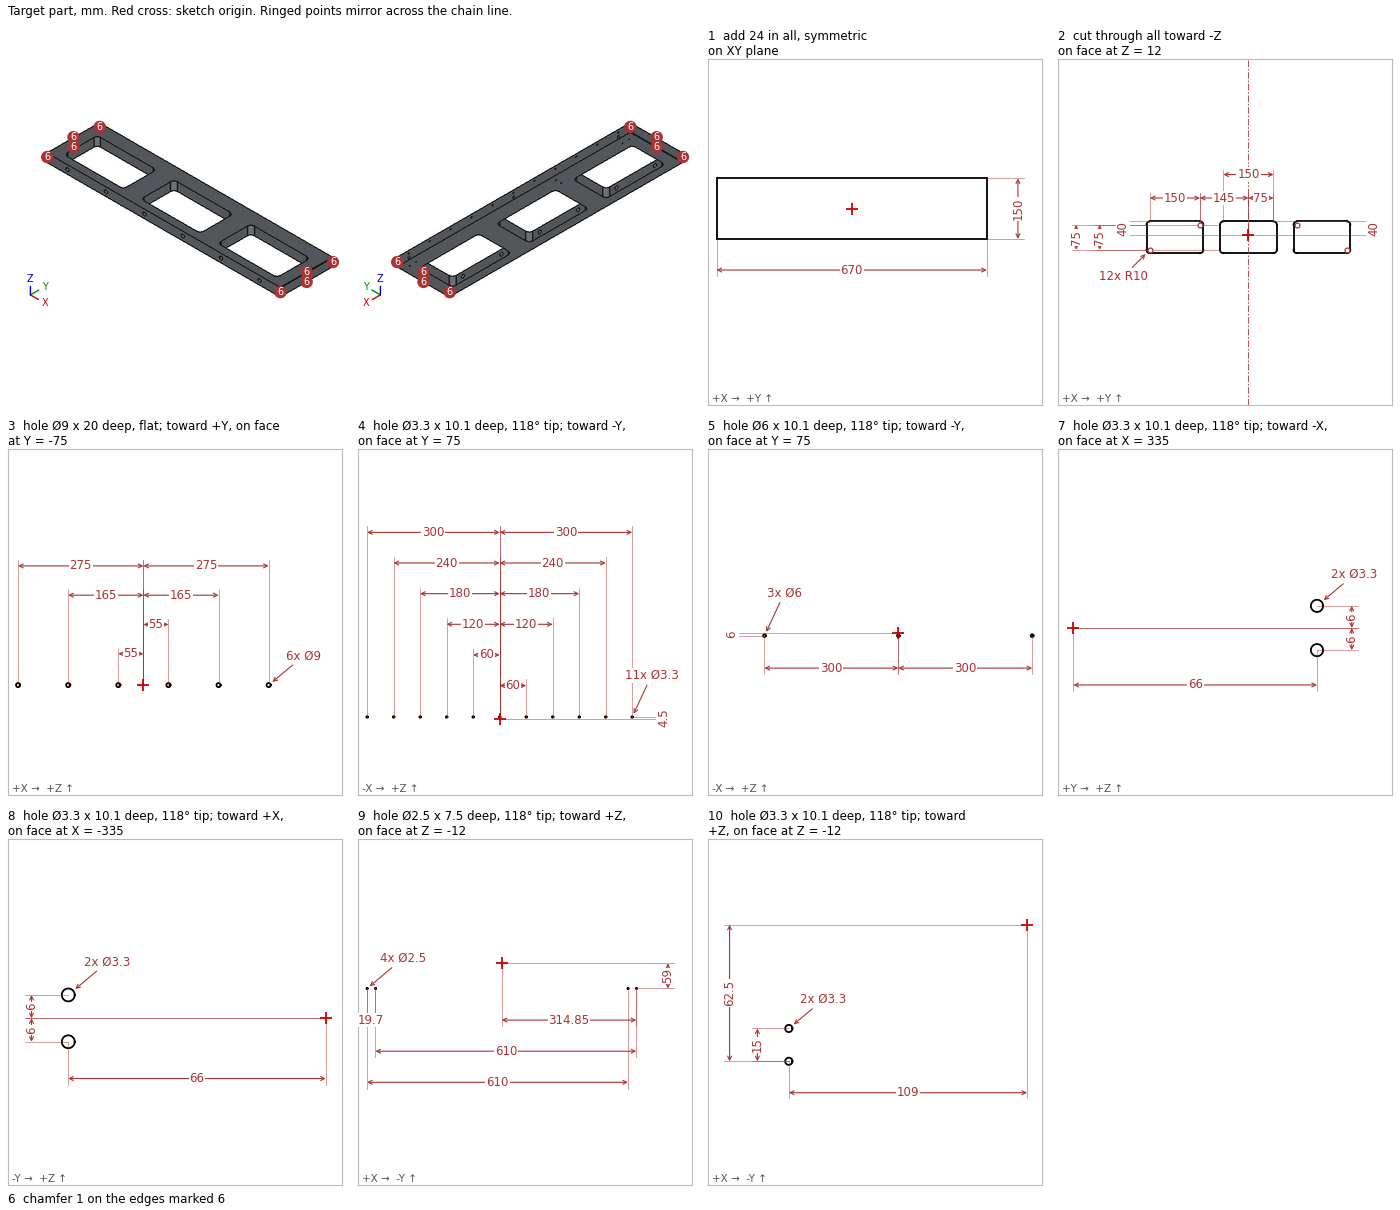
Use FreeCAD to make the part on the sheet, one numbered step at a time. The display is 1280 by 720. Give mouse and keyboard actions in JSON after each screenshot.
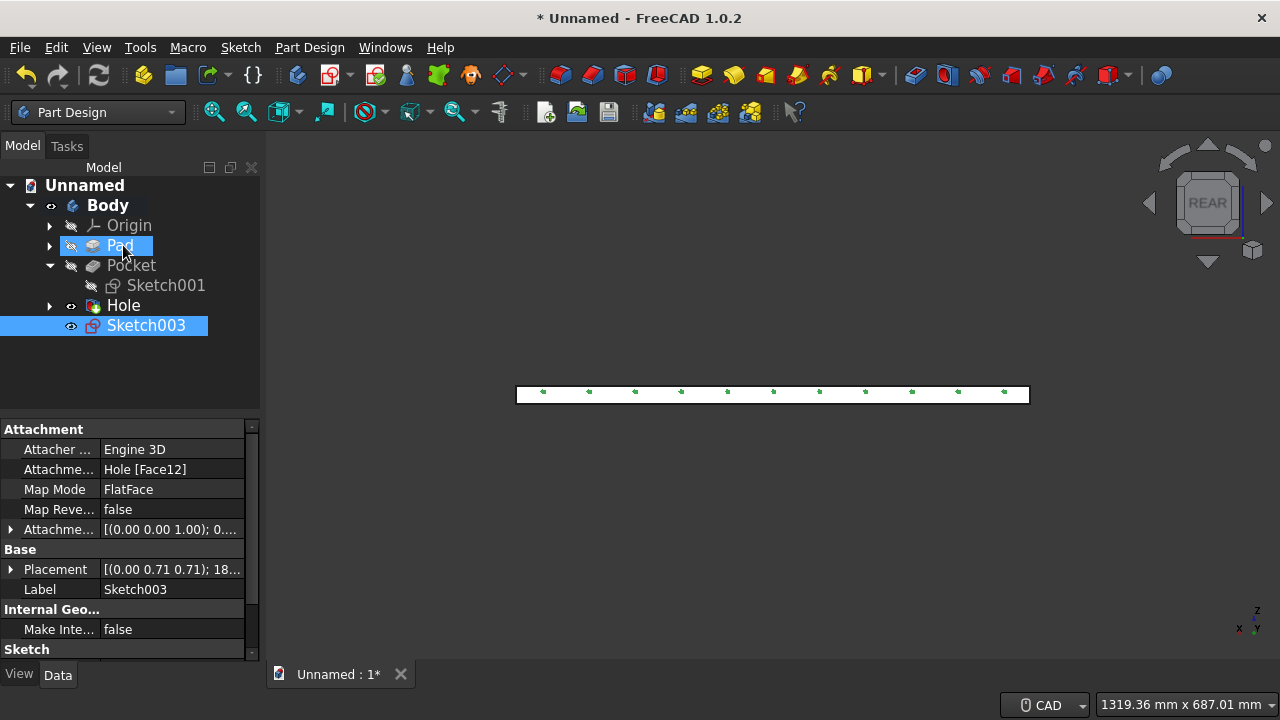
{"action": "left_click", "coordinate": [948, 76]}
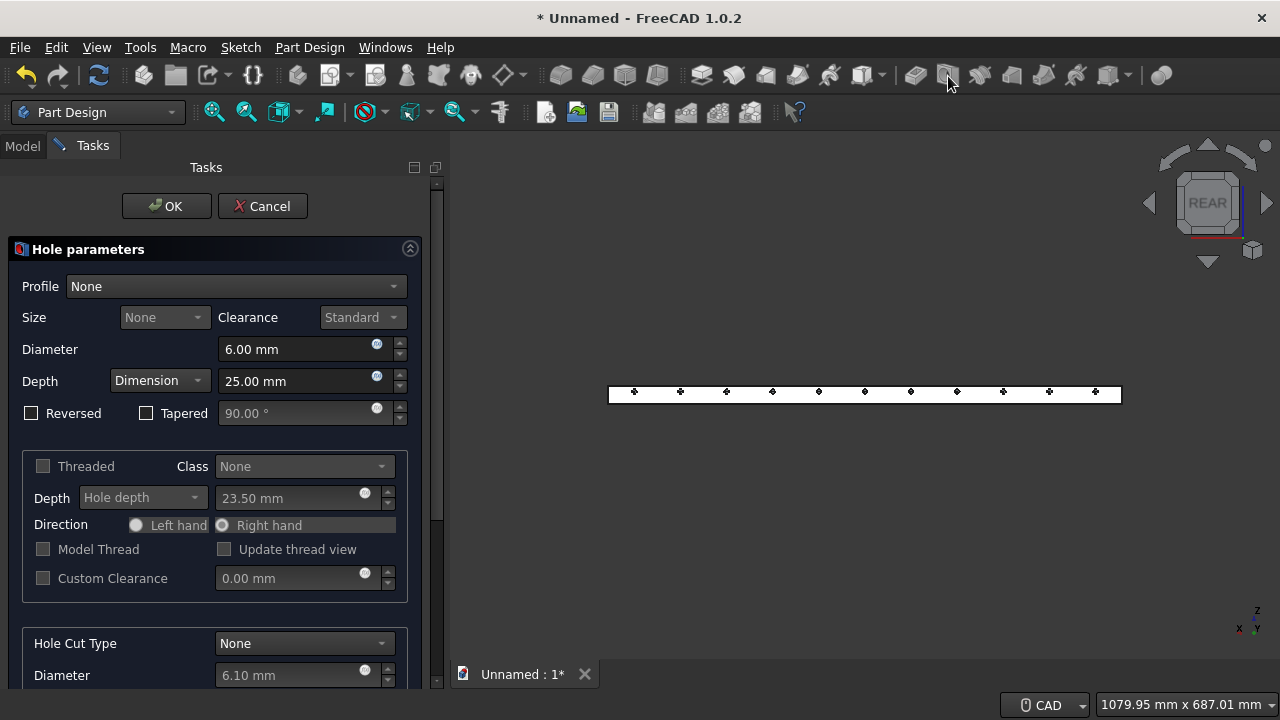
{"action": "triple_click", "coordinate": [305, 349]}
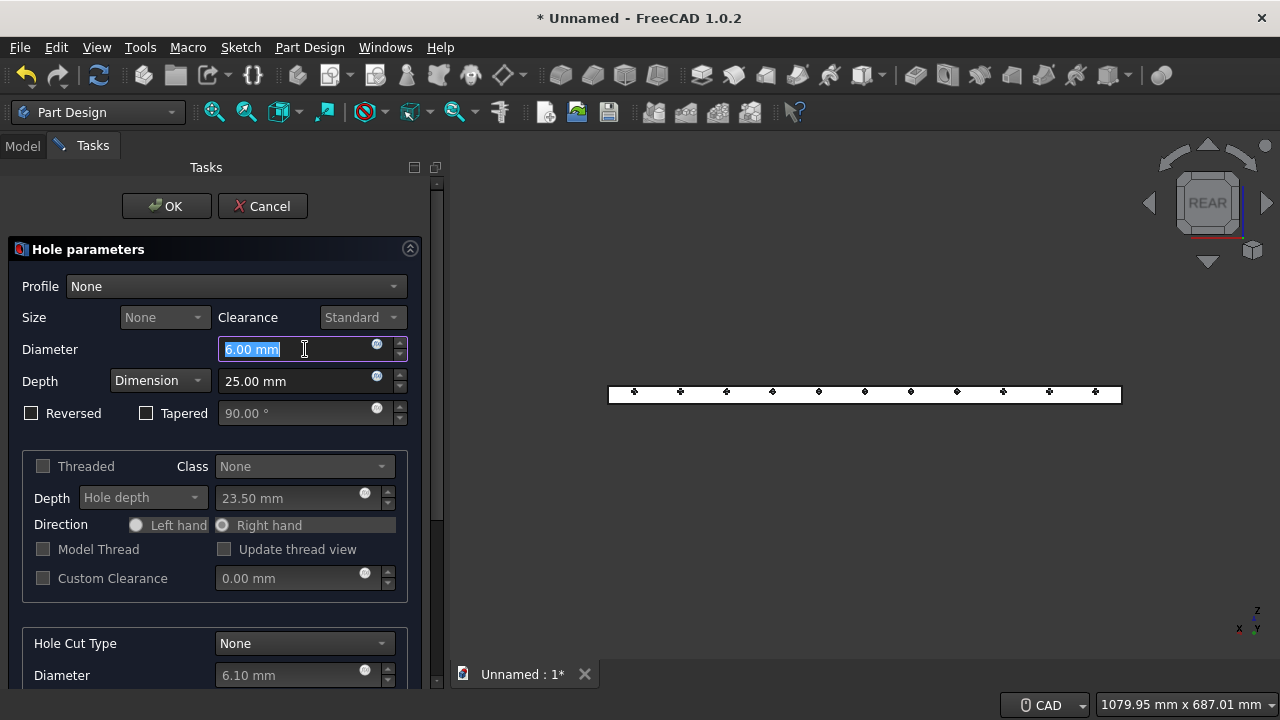
{"action": "type", "text": "3.3"}
{"action": "key", "text": "Tab"}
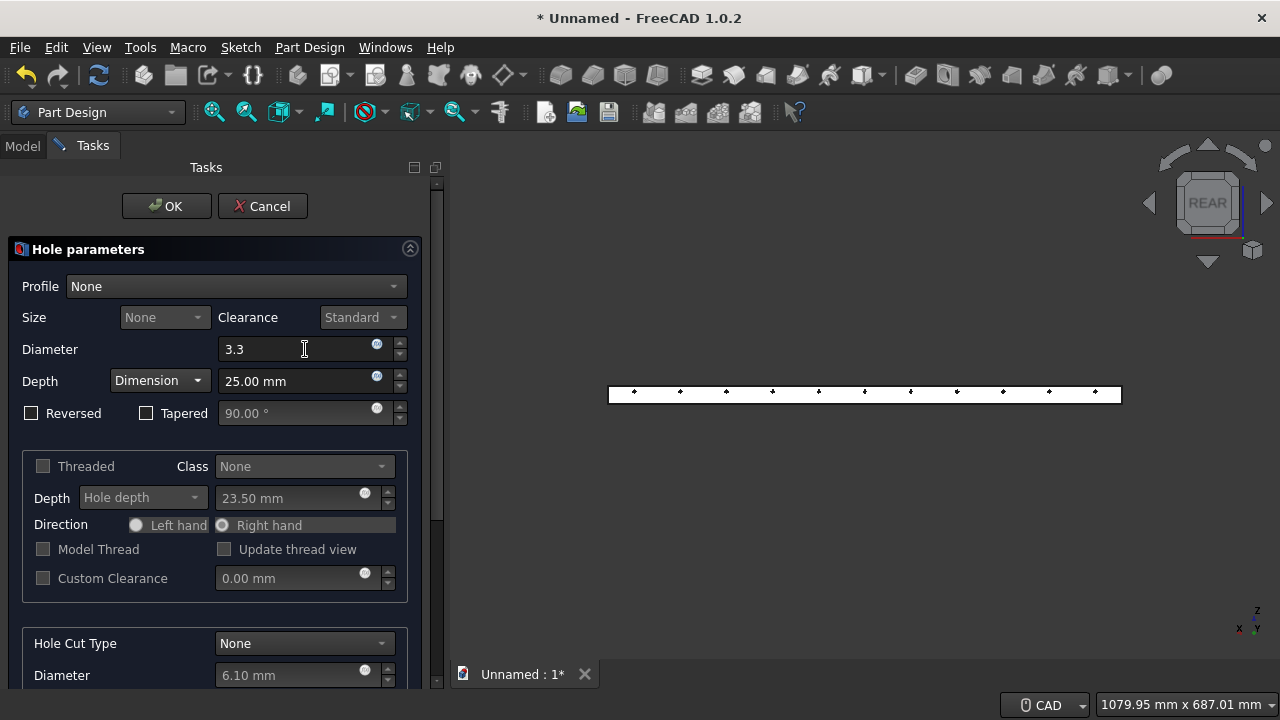
{"action": "triple_click", "coordinate": [305, 381]}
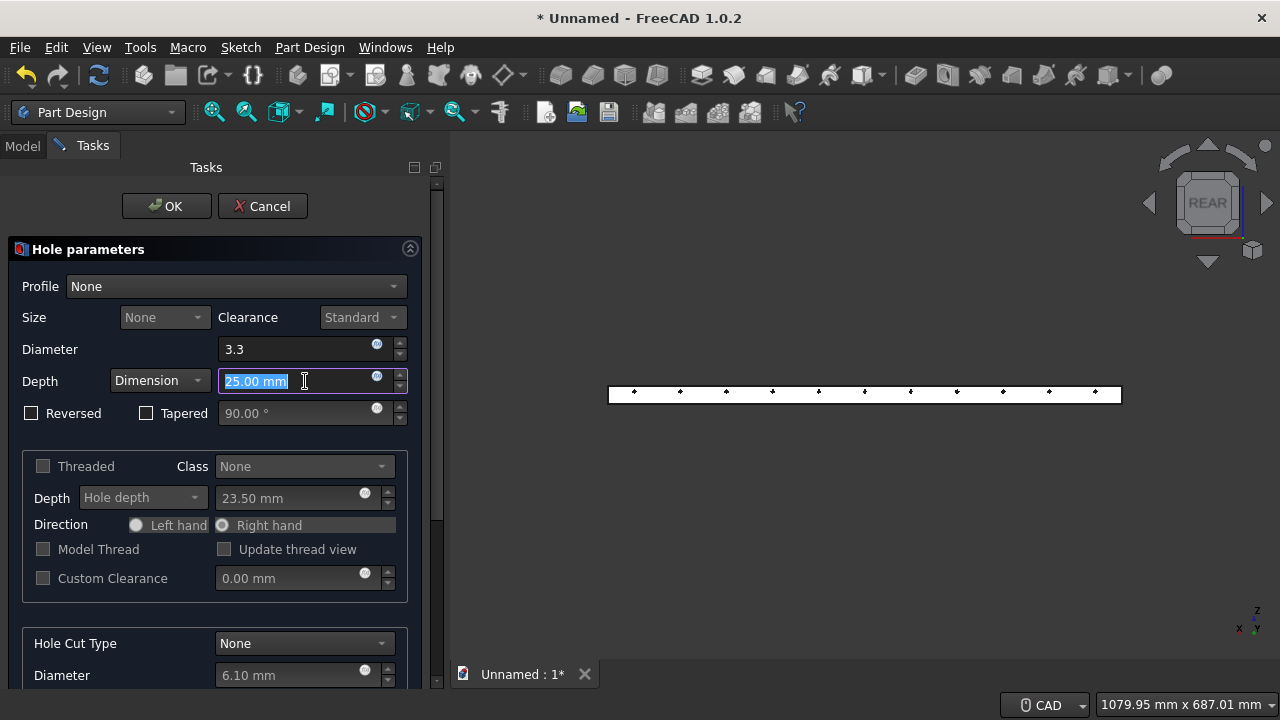
{"action": "type", "text": "10.1"}
{"action": "key", "text": "Tab"}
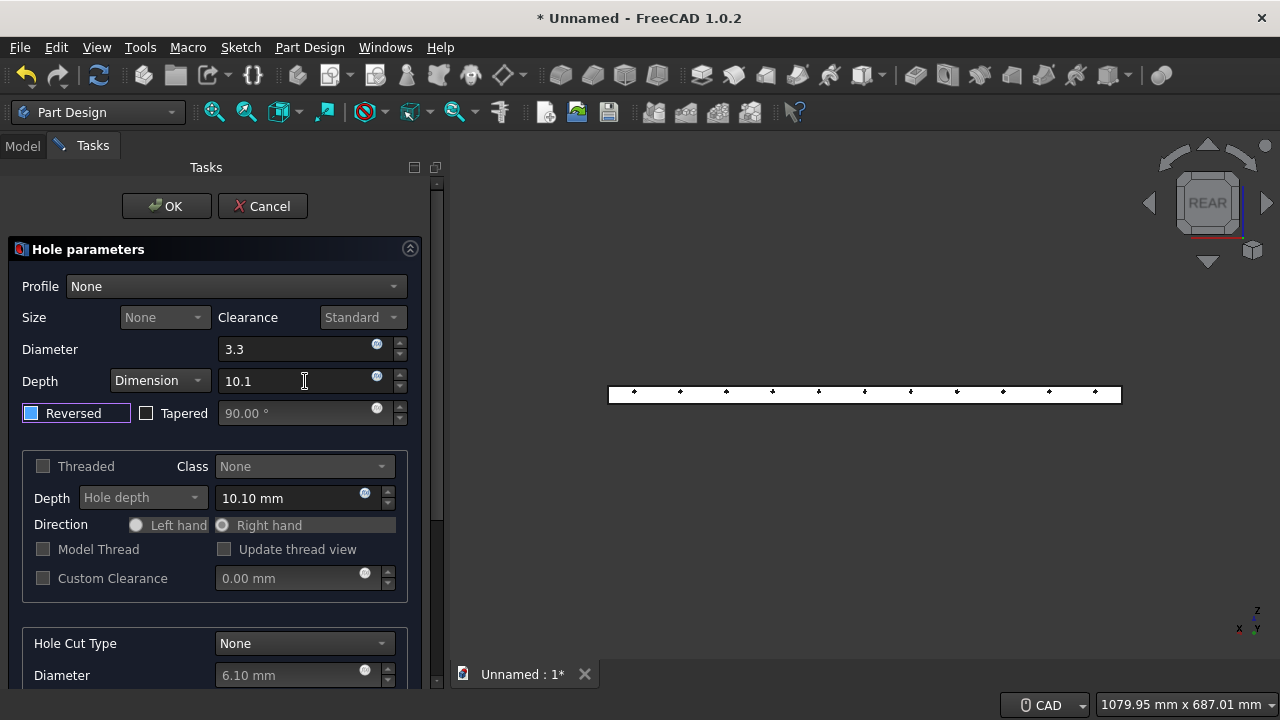
{"action": "left_click", "coordinate": [167, 206]}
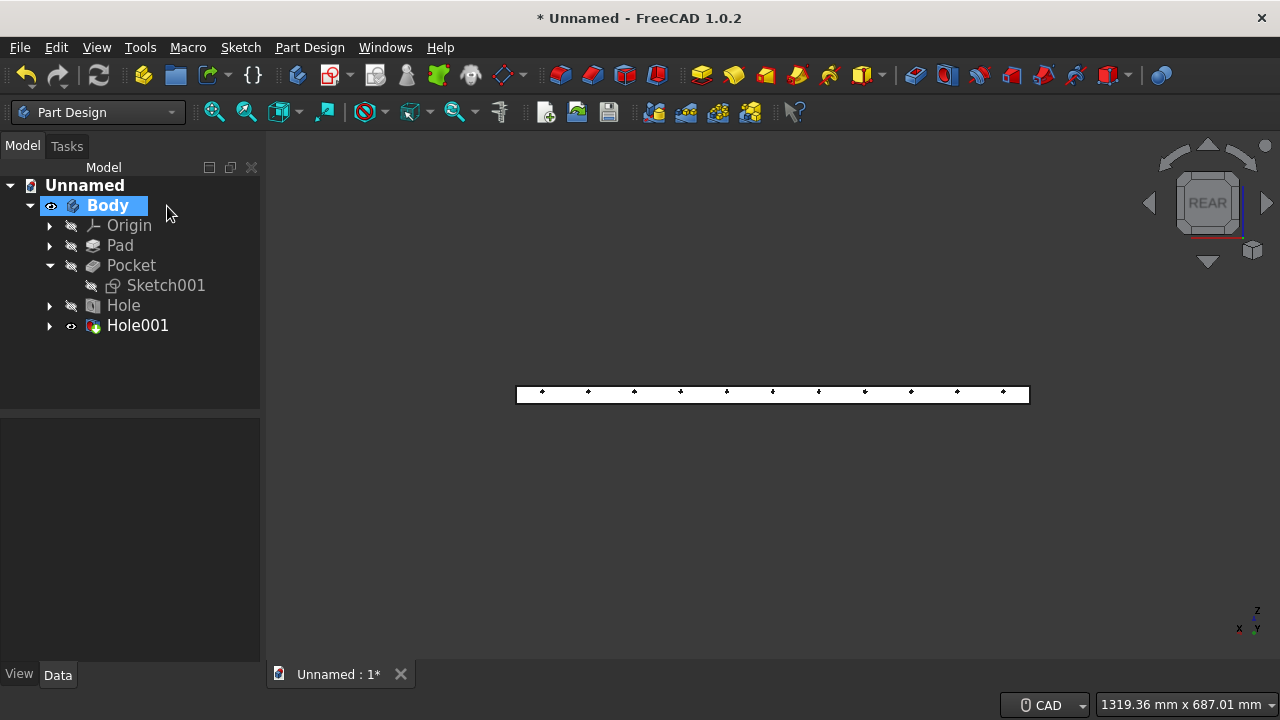
{"action": "left_click", "coordinate": [699, 394]}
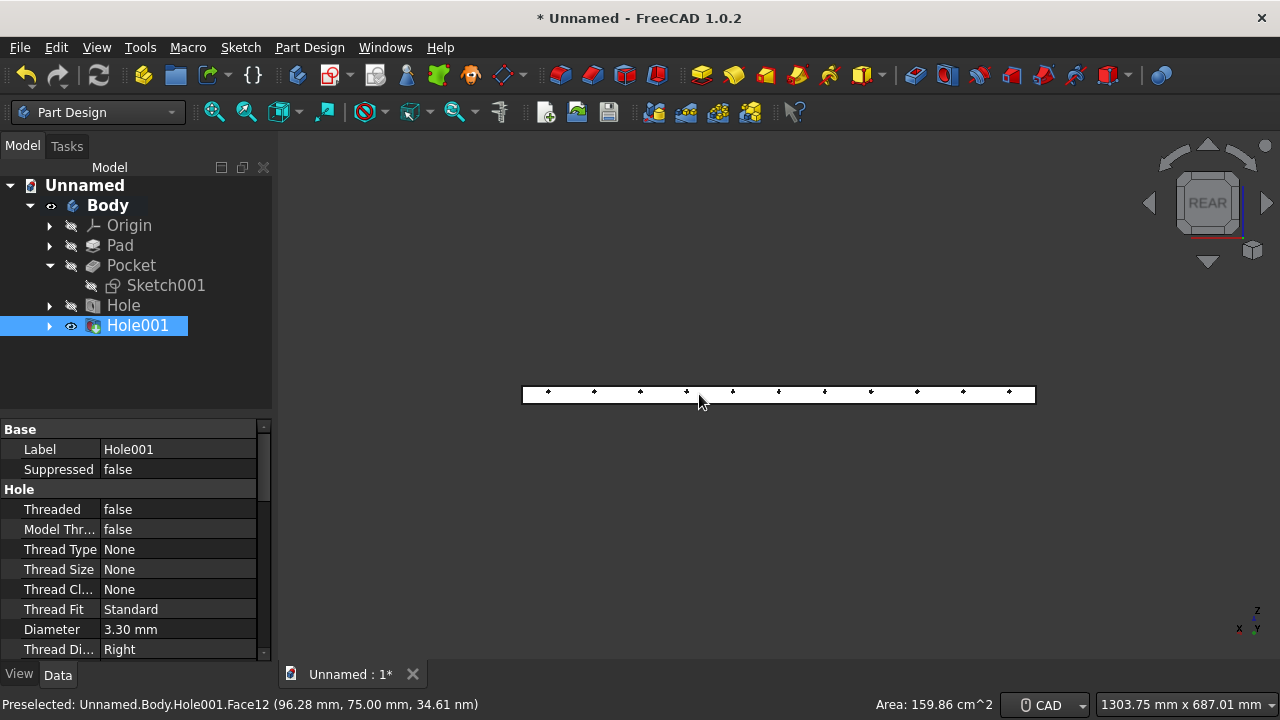
{"action": "left_click", "coordinate": [330, 76]}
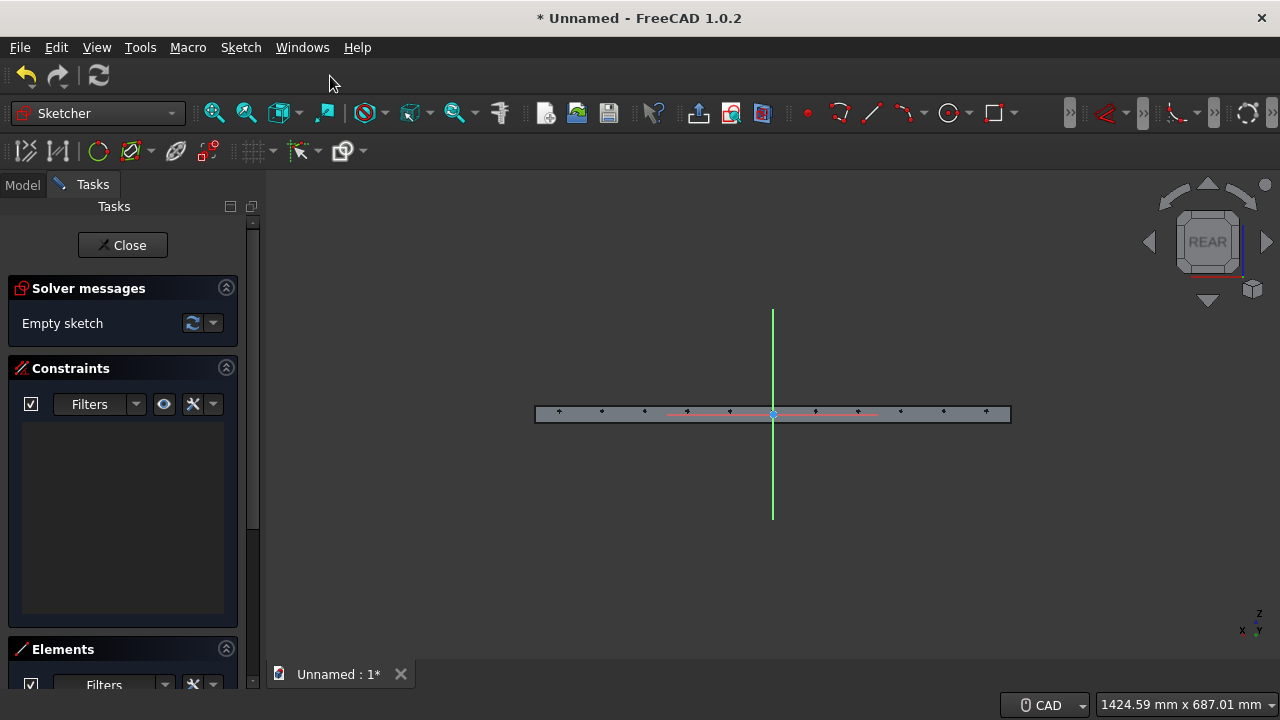
{"action": "key", "text": "g c"}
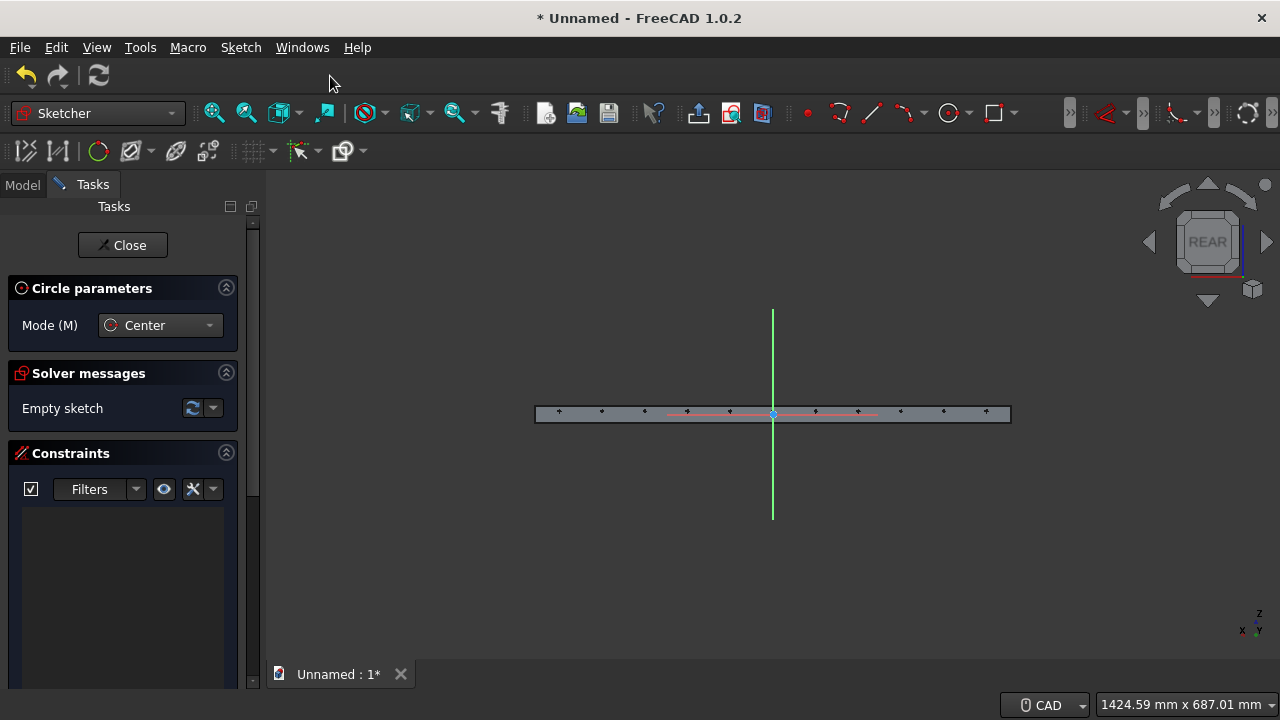
{"action": "scroll", "coordinate": [559, 419], "scroll_direction": "up", "scroll_amount": 12}